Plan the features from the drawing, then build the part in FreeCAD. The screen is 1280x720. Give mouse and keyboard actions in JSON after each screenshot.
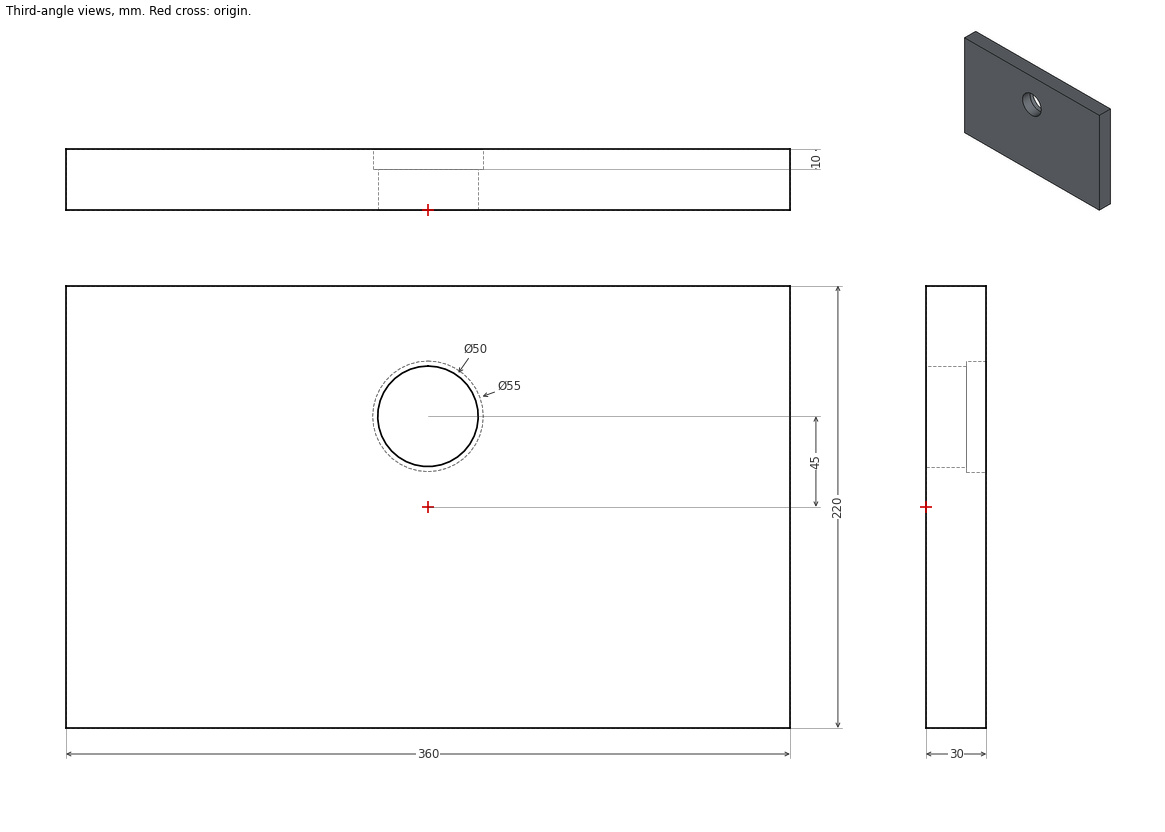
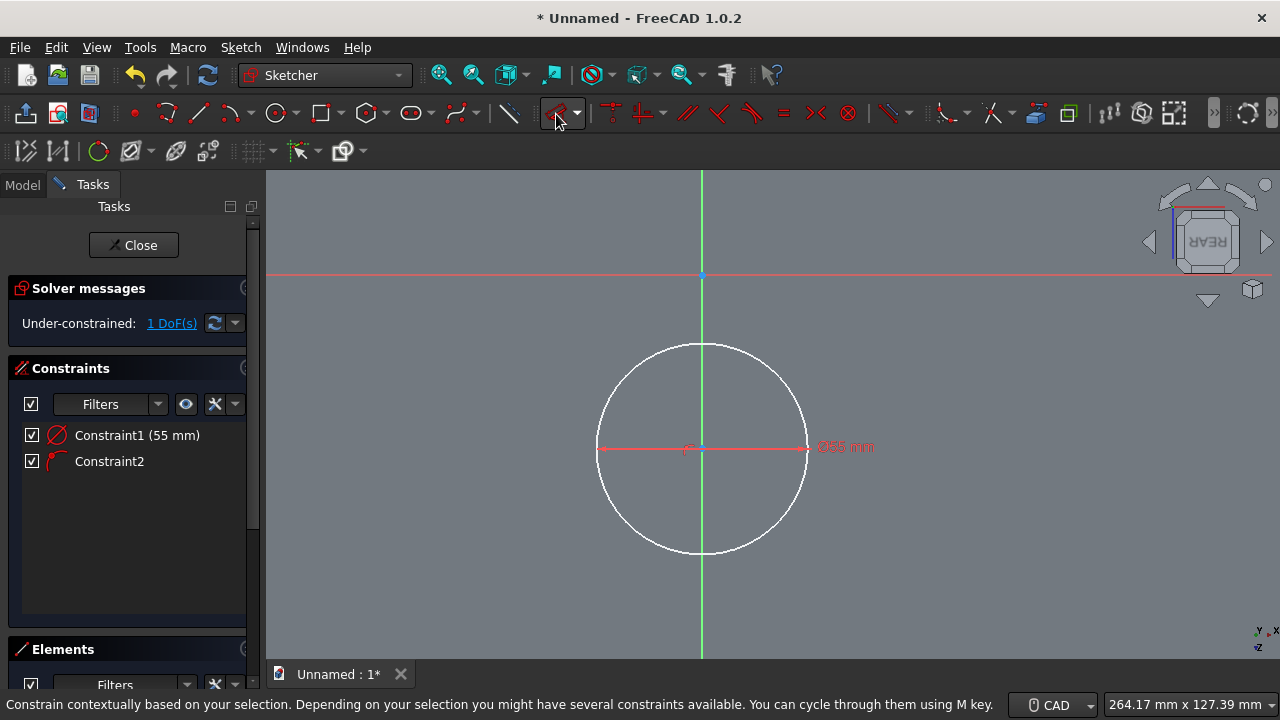
{"action": "left_click", "coordinate": [702, 449]}
{"action": "left_click", "coordinate": [736, 322]}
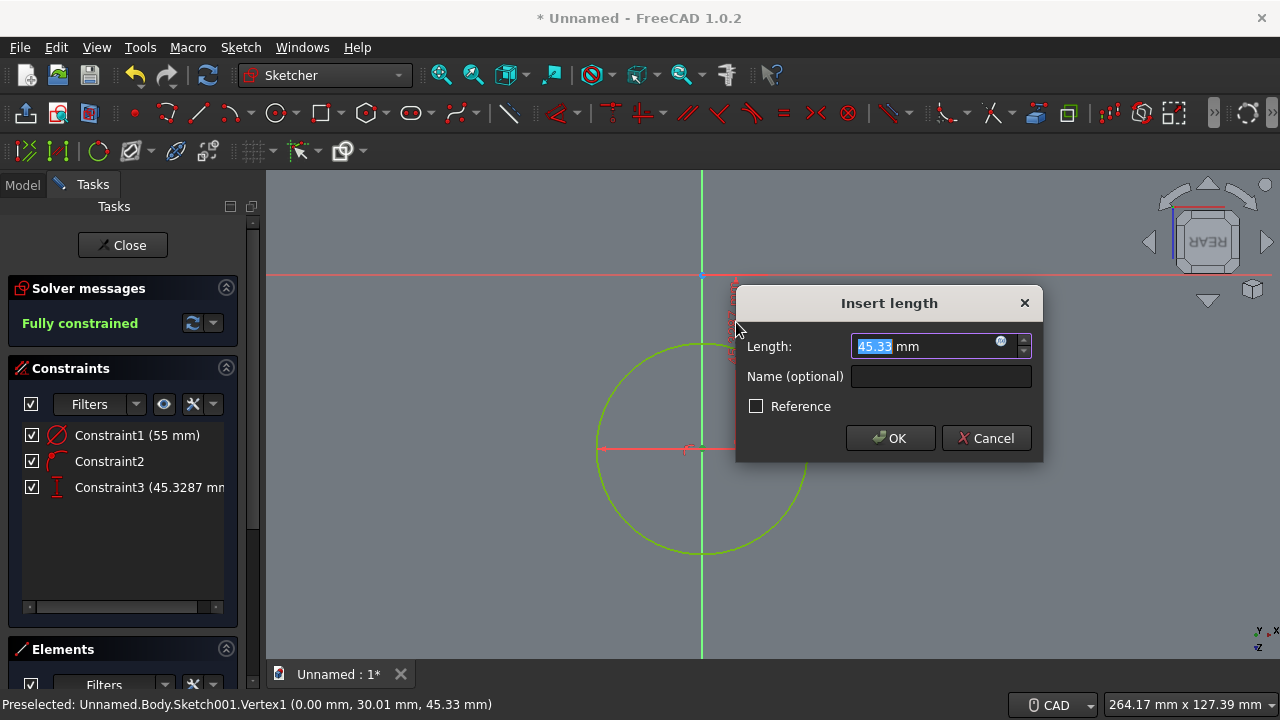
{"action": "type", "text": "45"}
{"action": "key", "text": "Return"}
{"action": "key", "text": "Escape"}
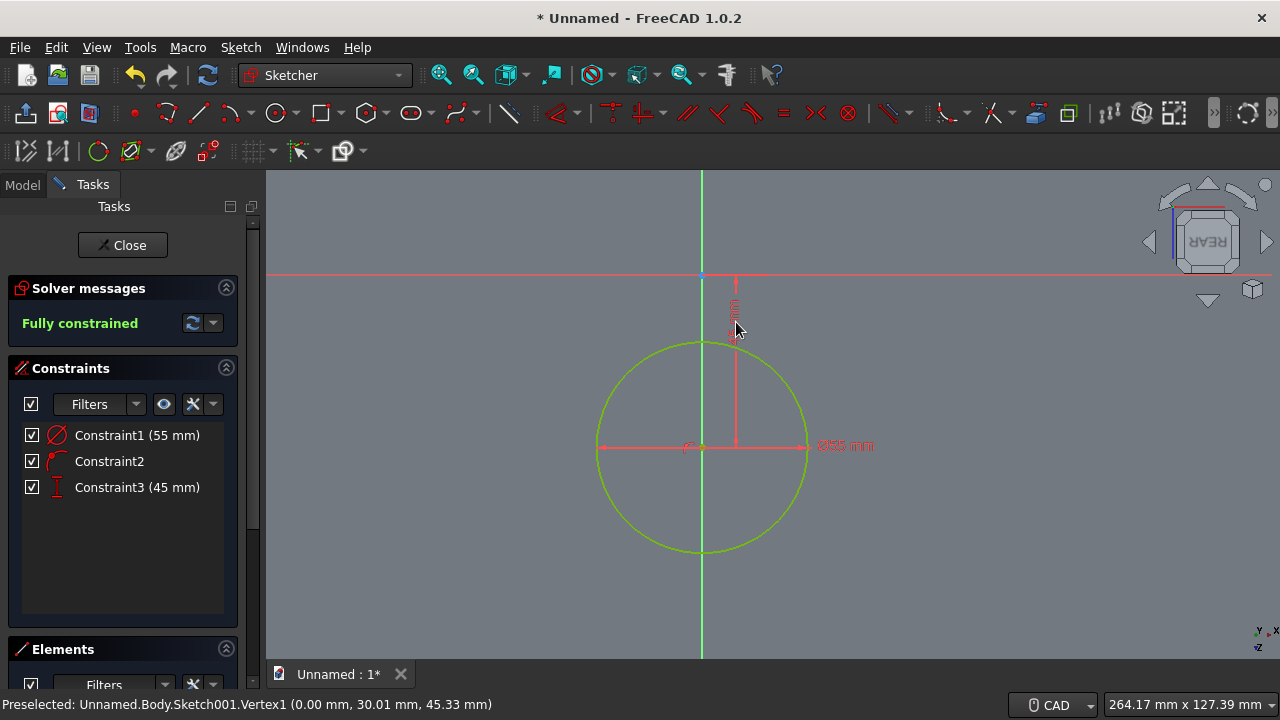
{"action": "left_click", "coordinate": [123, 245]}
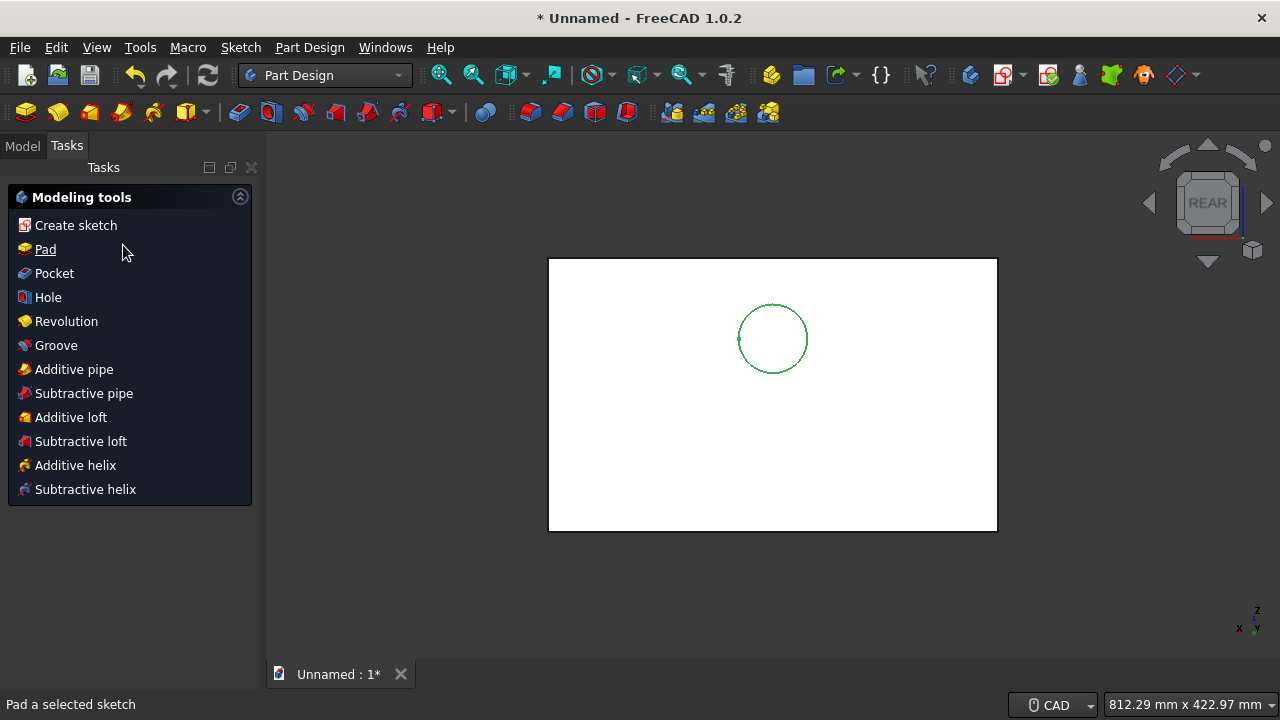
{"action": "left_click", "coordinate": [240, 112]}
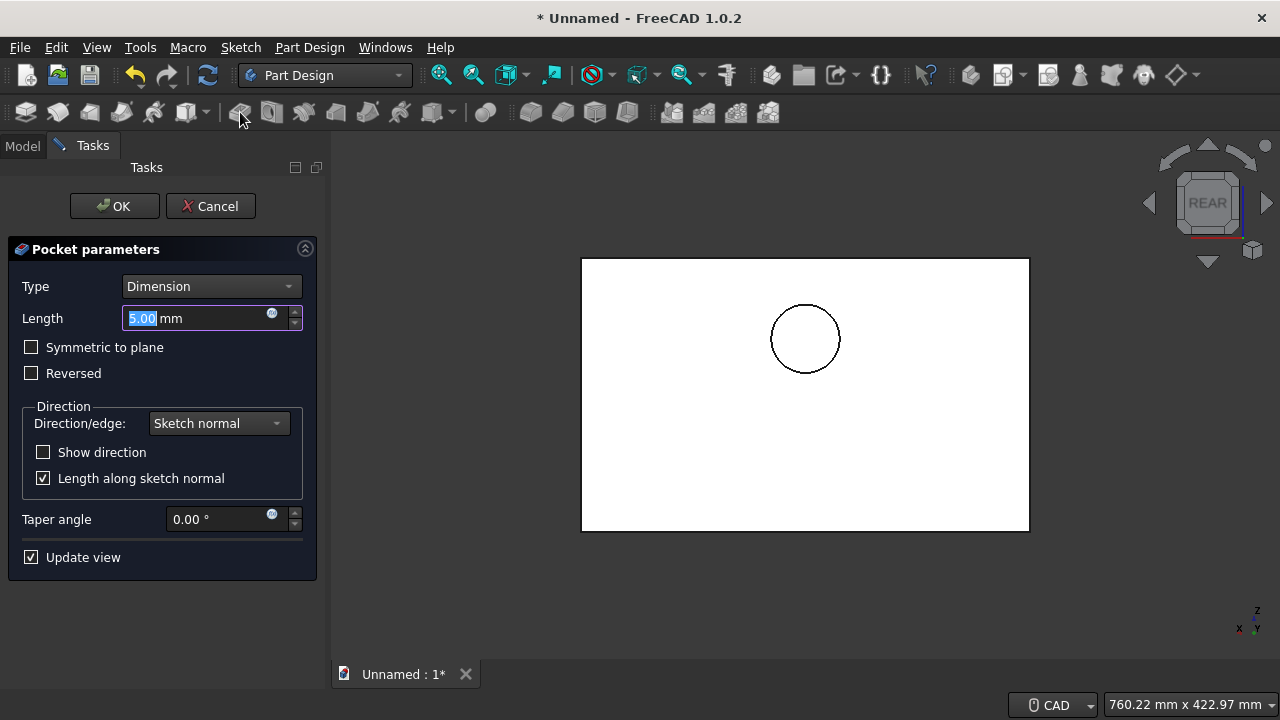
{"action": "type", "text": "10"}
{"action": "key", "text": "Tab"}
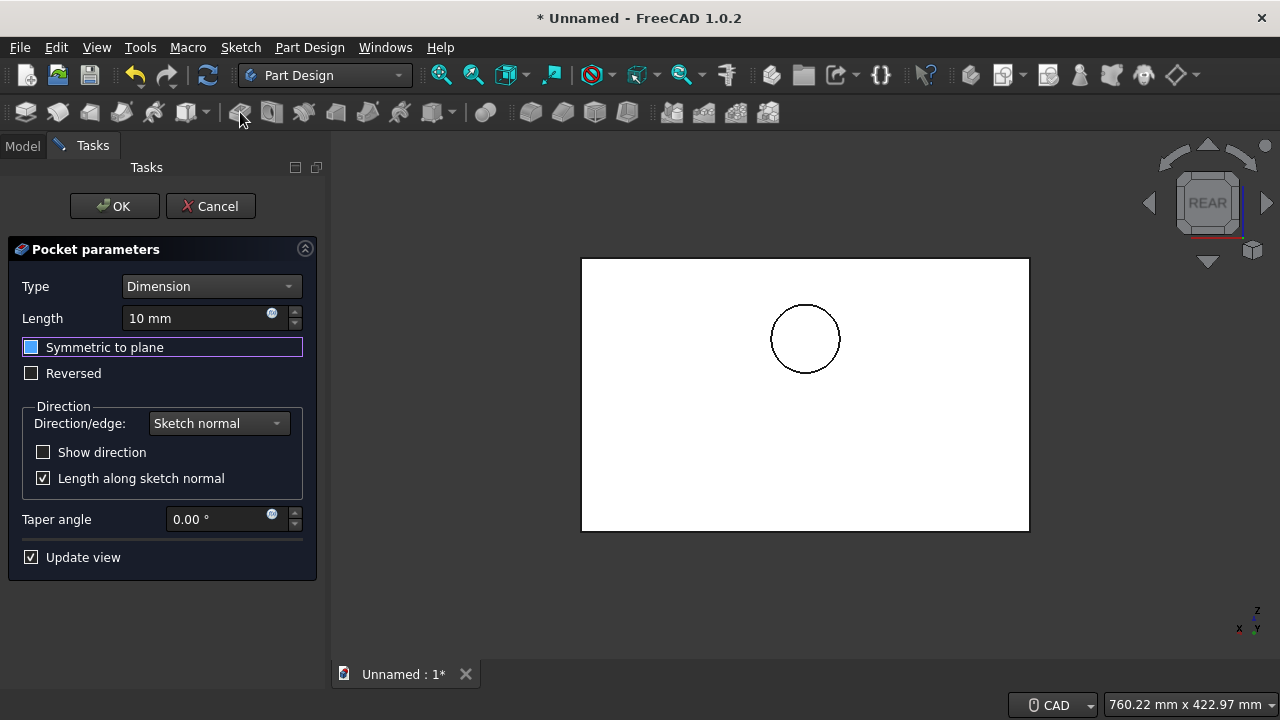
{"action": "left_click", "coordinate": [115, 206]}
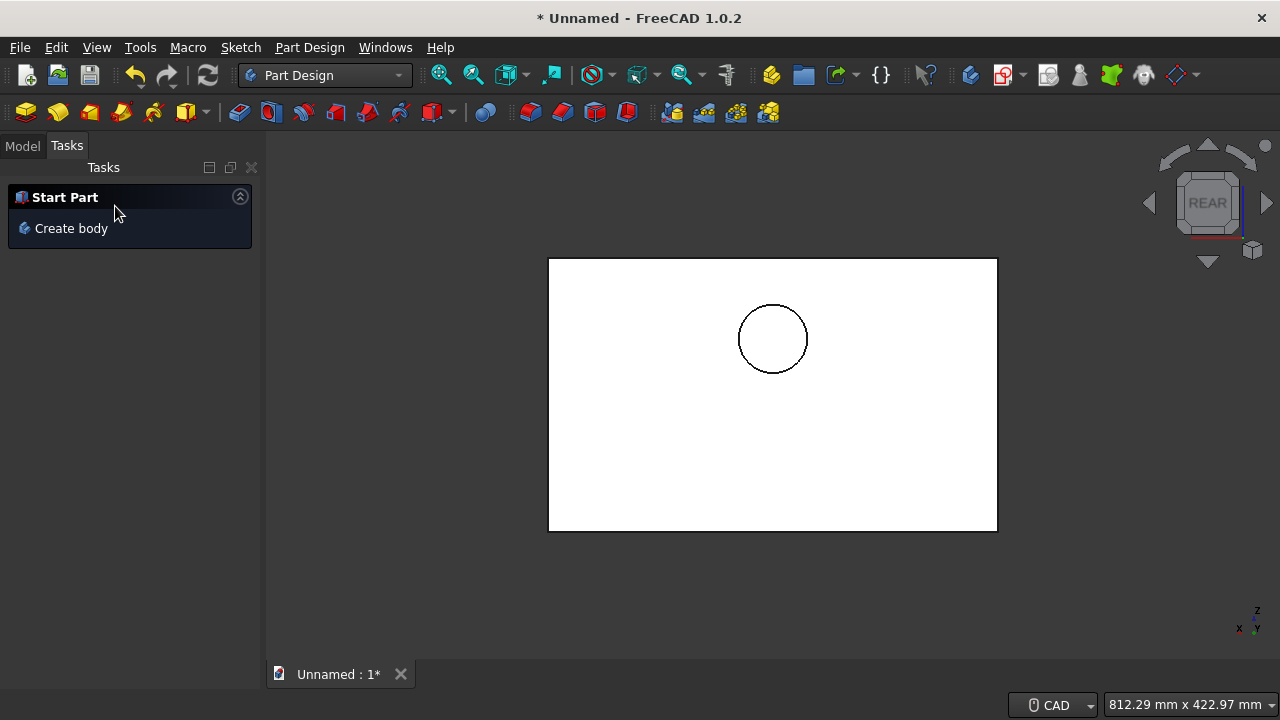
{"action": "left_click", "coordinate": [645, 394]}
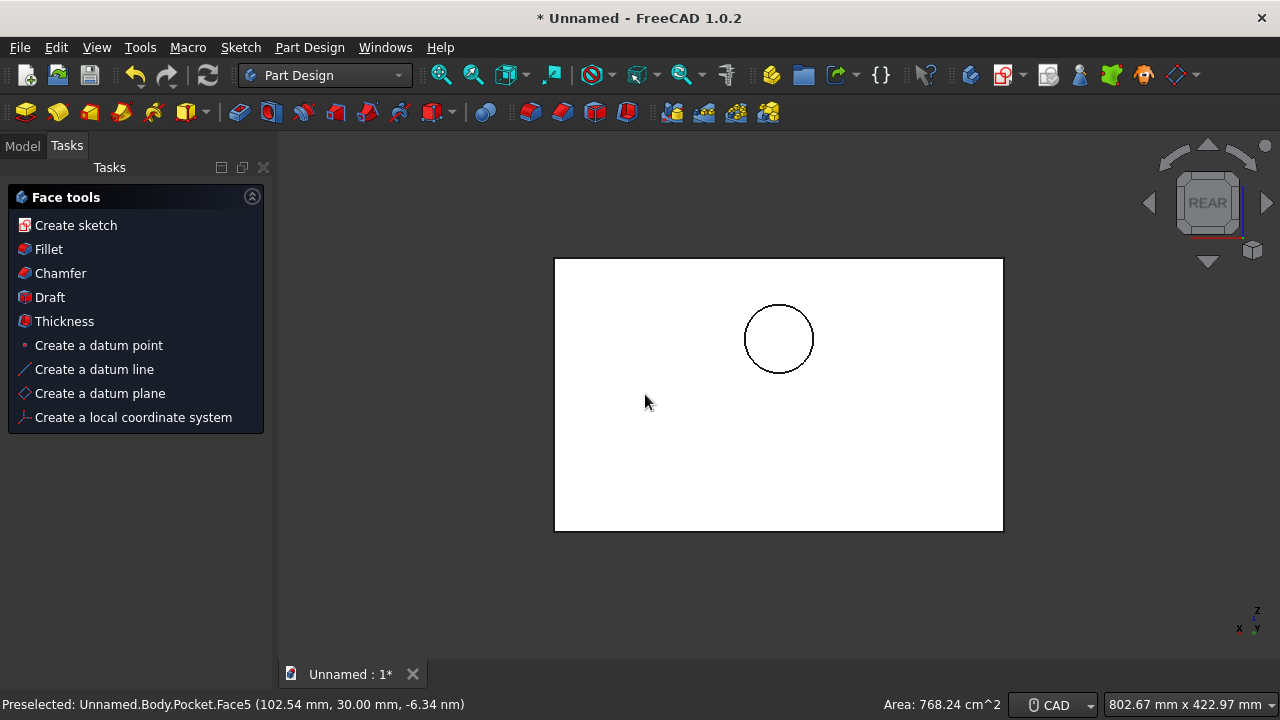
{"action": "left_click", "coordinate": [1004, 76]}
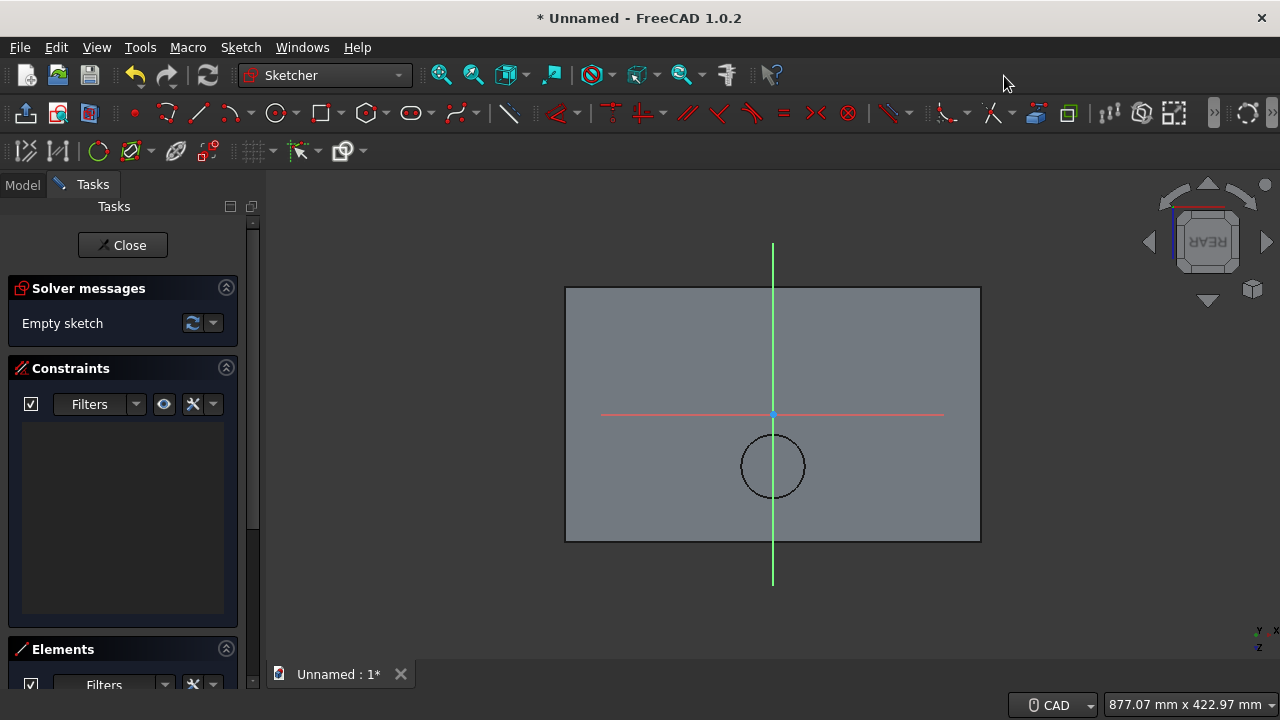
{"action": "scroll", "coordinate": [795, 468], "scroll_direction": "up", "scroll_amount": 7}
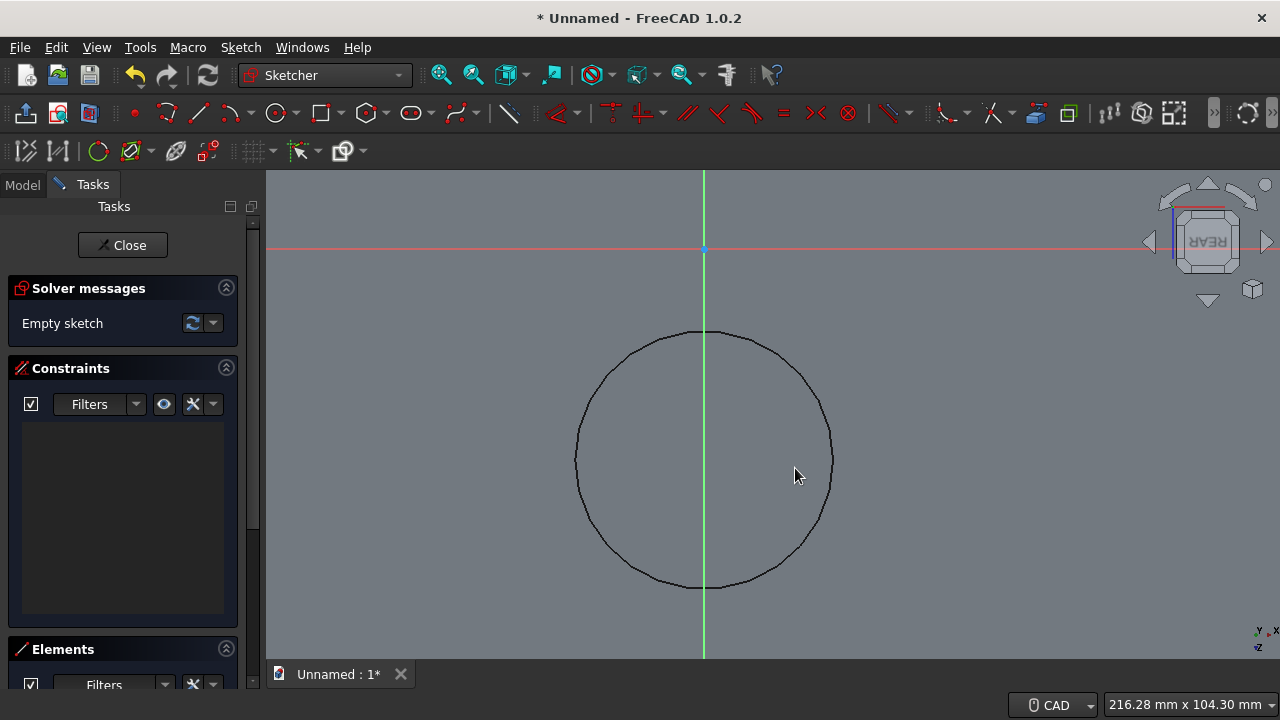
{"action": "left_click", "coordinate": [276, 114]}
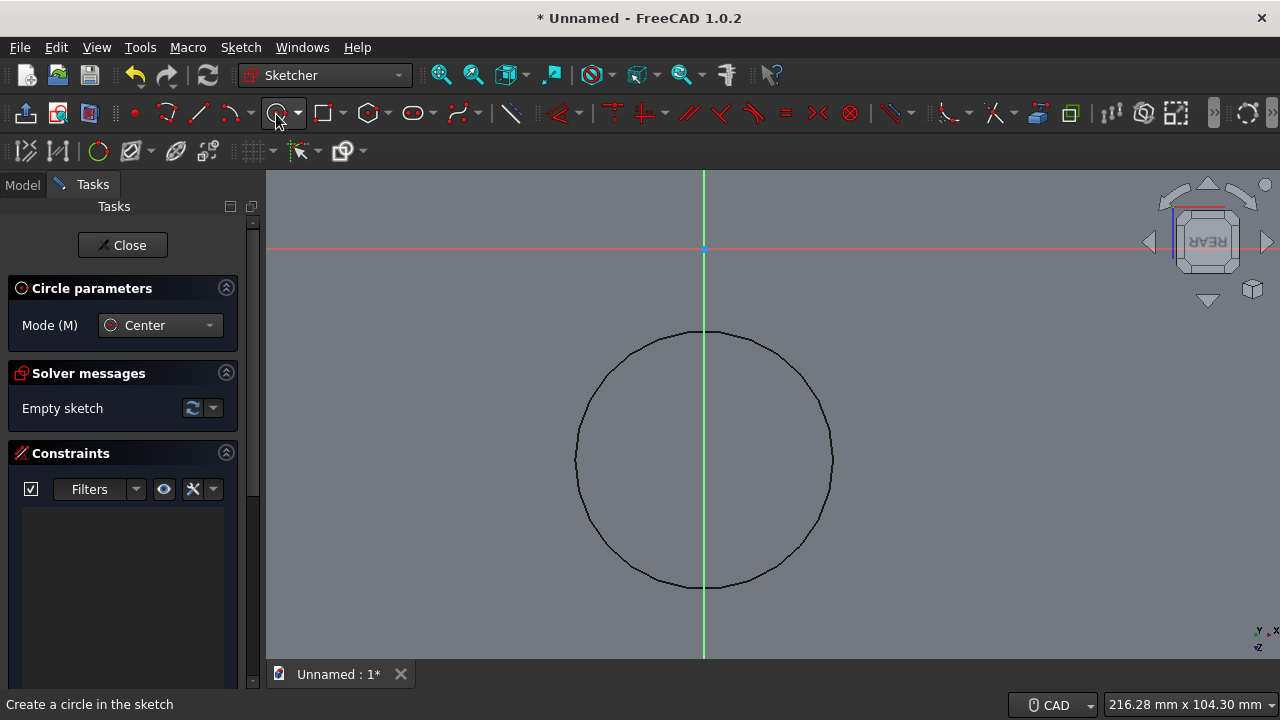
{"action": "left_click", "coordinate": [704, 460]}
{"action": "mouse_move", "coordinate": [787, 377]}